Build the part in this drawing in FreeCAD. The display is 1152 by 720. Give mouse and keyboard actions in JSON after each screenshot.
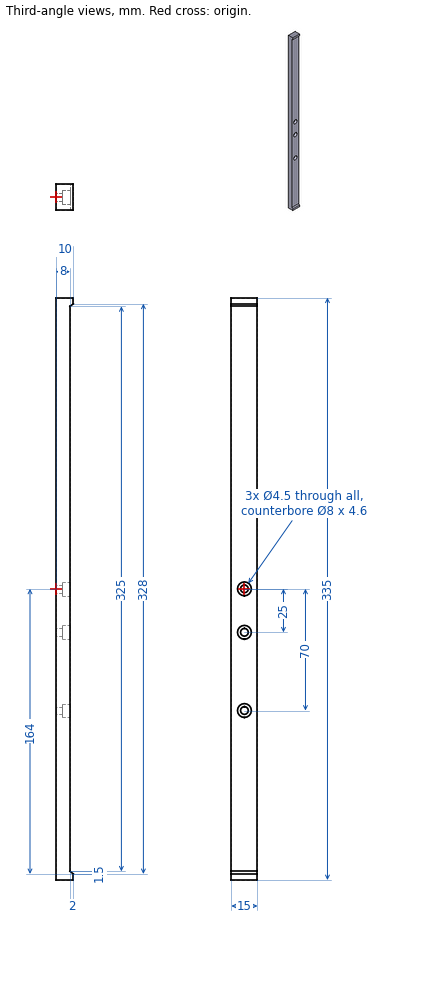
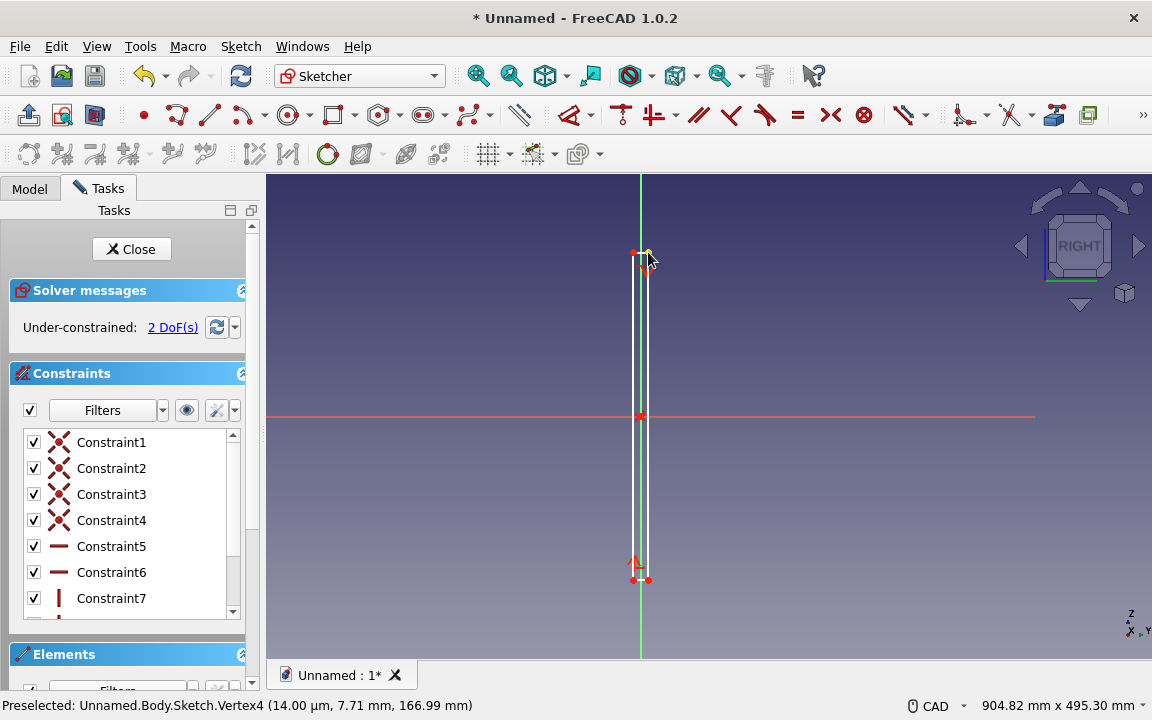
{"action": "scroll", "coordinate": [639, 580], "scroll_direction": "up", "scroll_amount": 5}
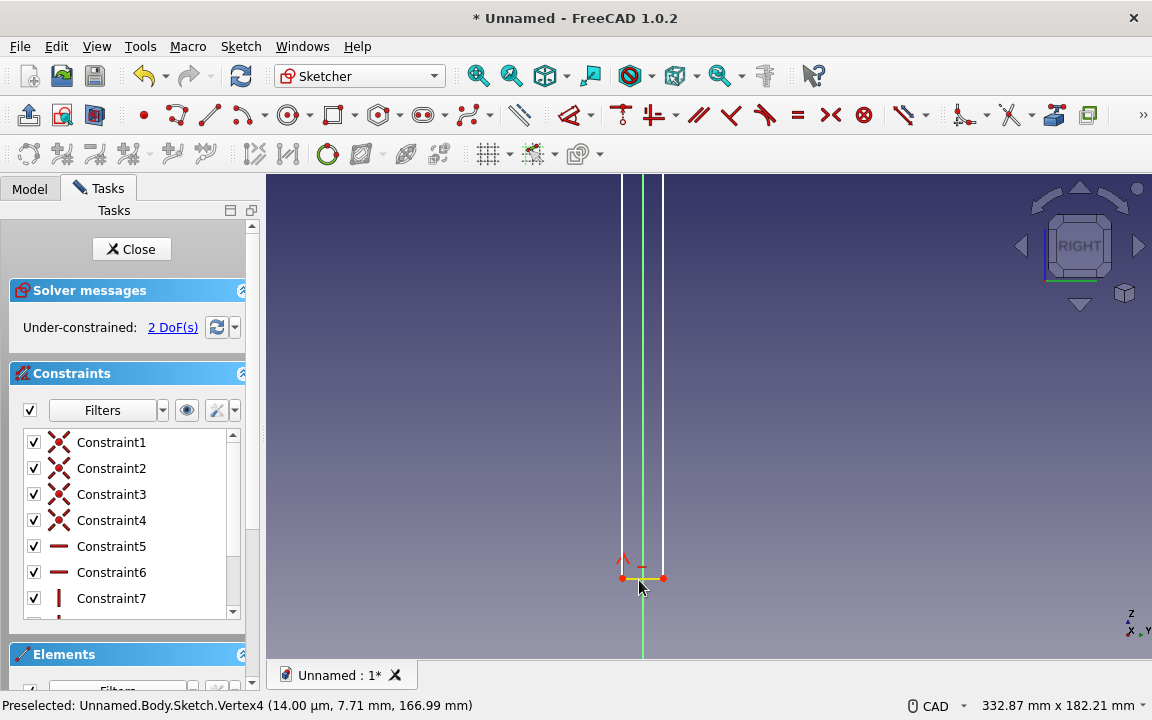
{"action": "left_click", "coordinate": [639, 579]}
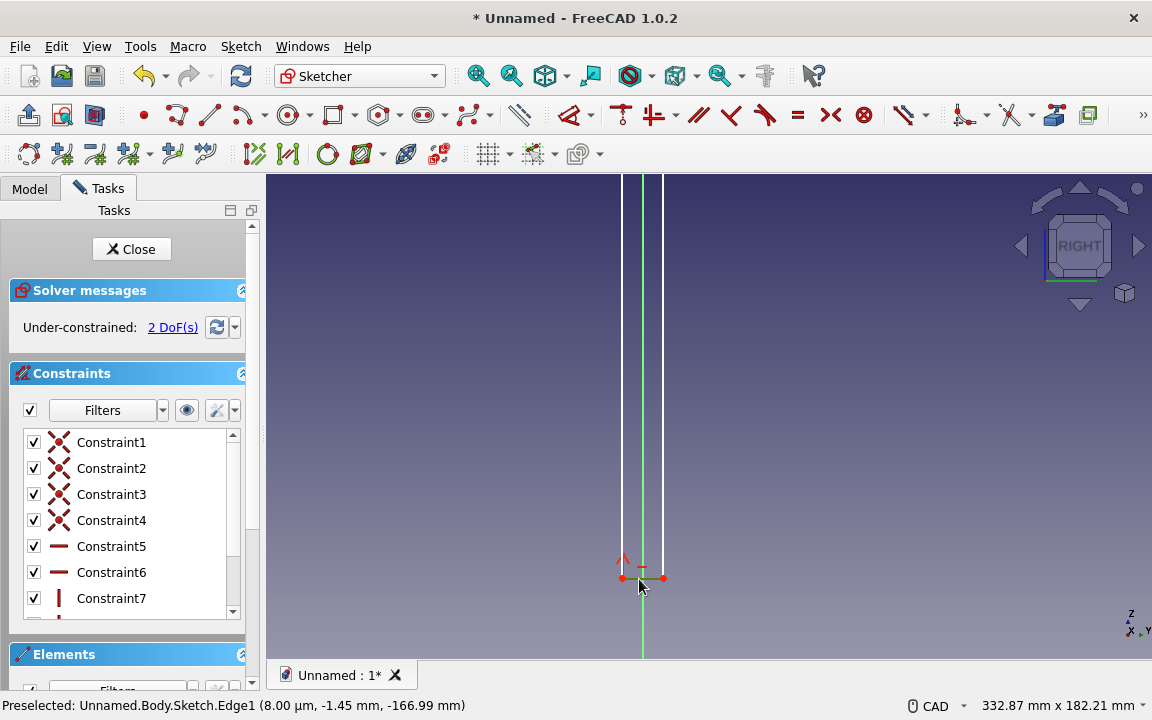
{"action": "key", "text": "l"}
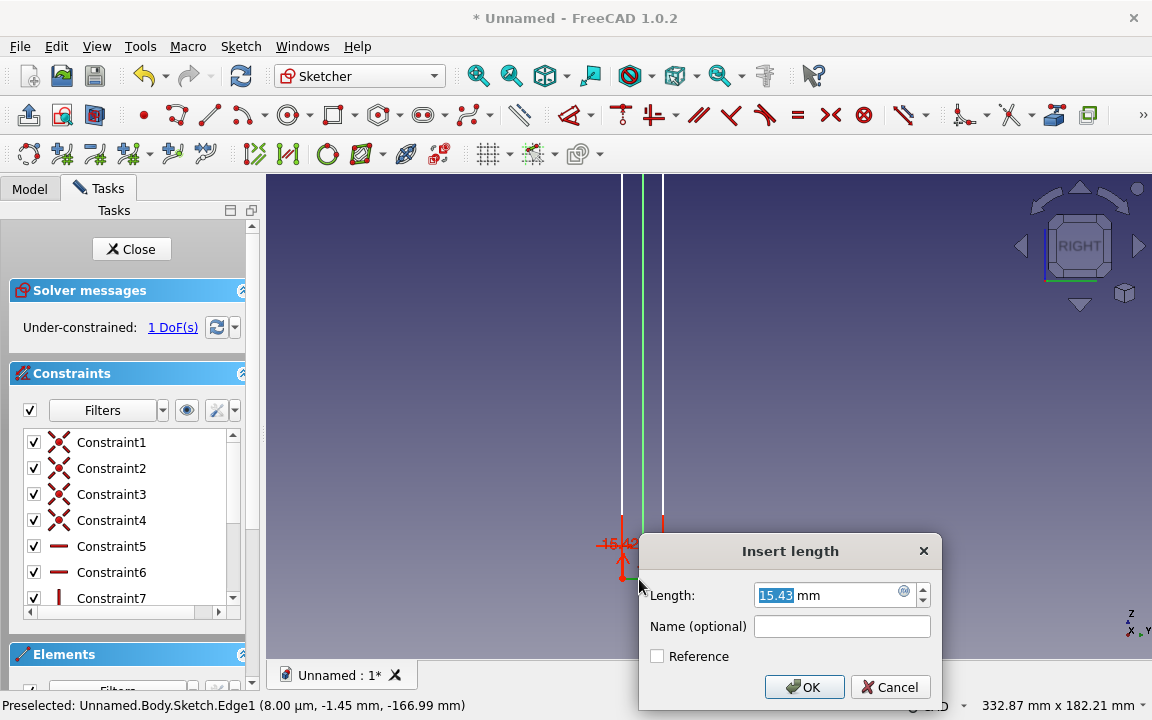
{"action": "type", "text": "15"}
{"action": "key", "text": "Return"}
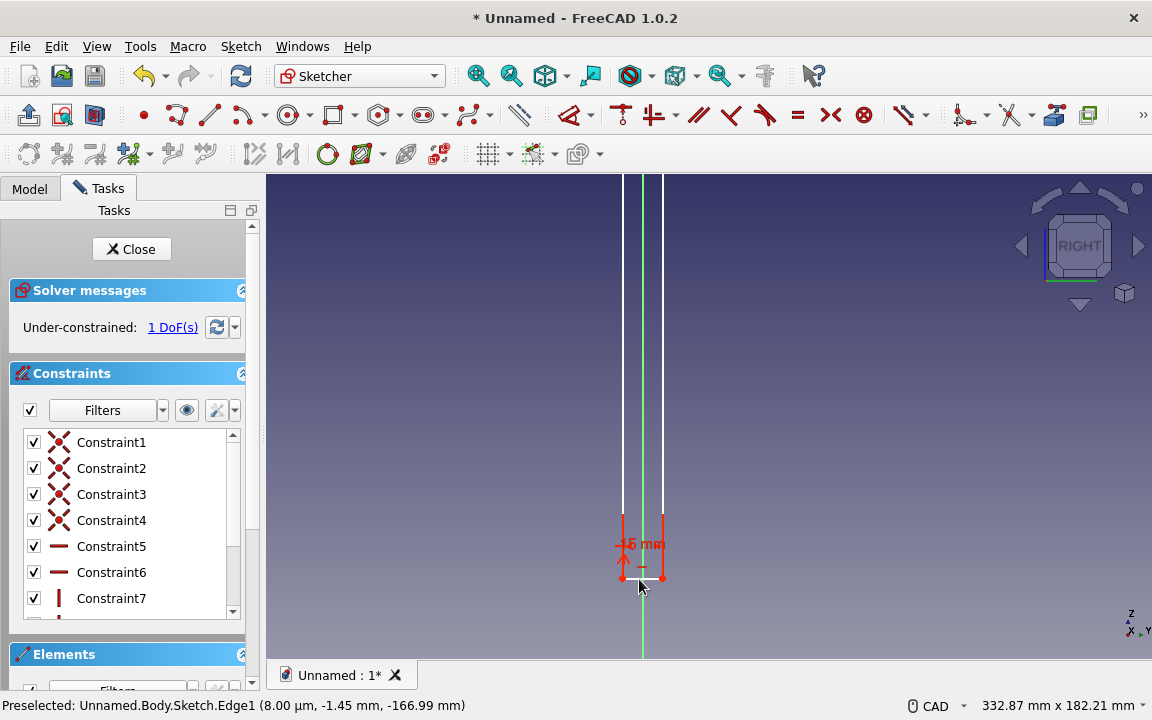
{"action": "left_click", "coordinate": [663, 312]}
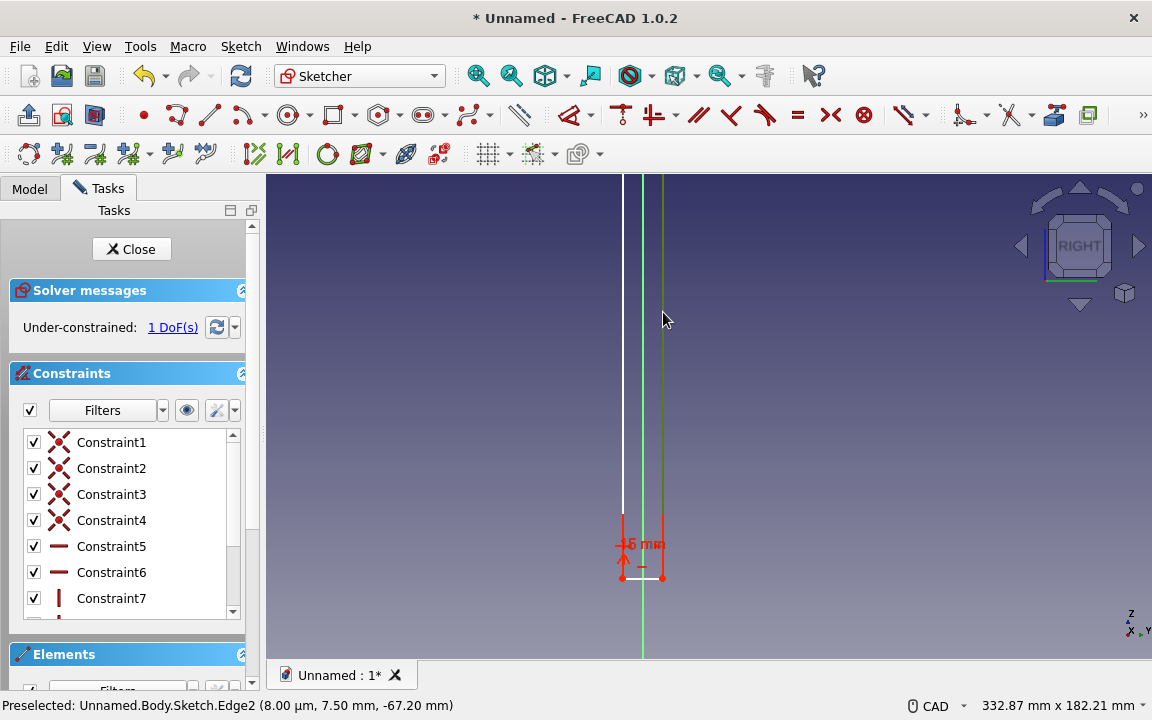
{"action": "key", "text": "i"}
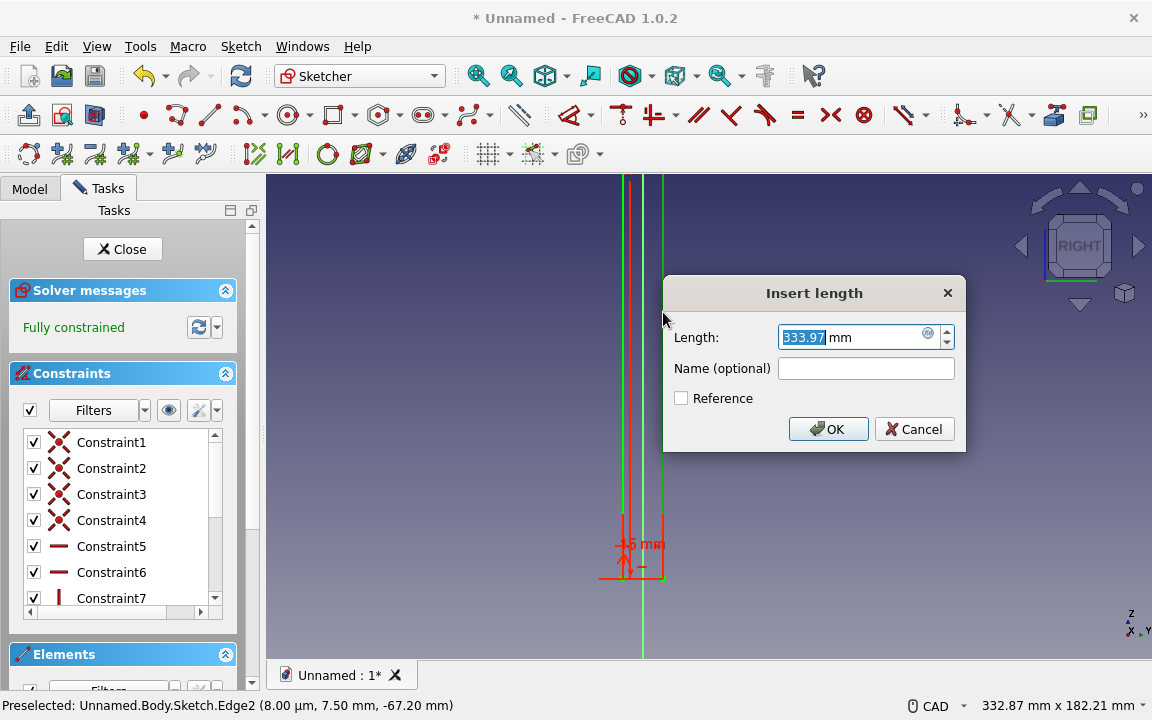
{"action": "type", "text": "335"}
{"action": "key", "text": "Return"}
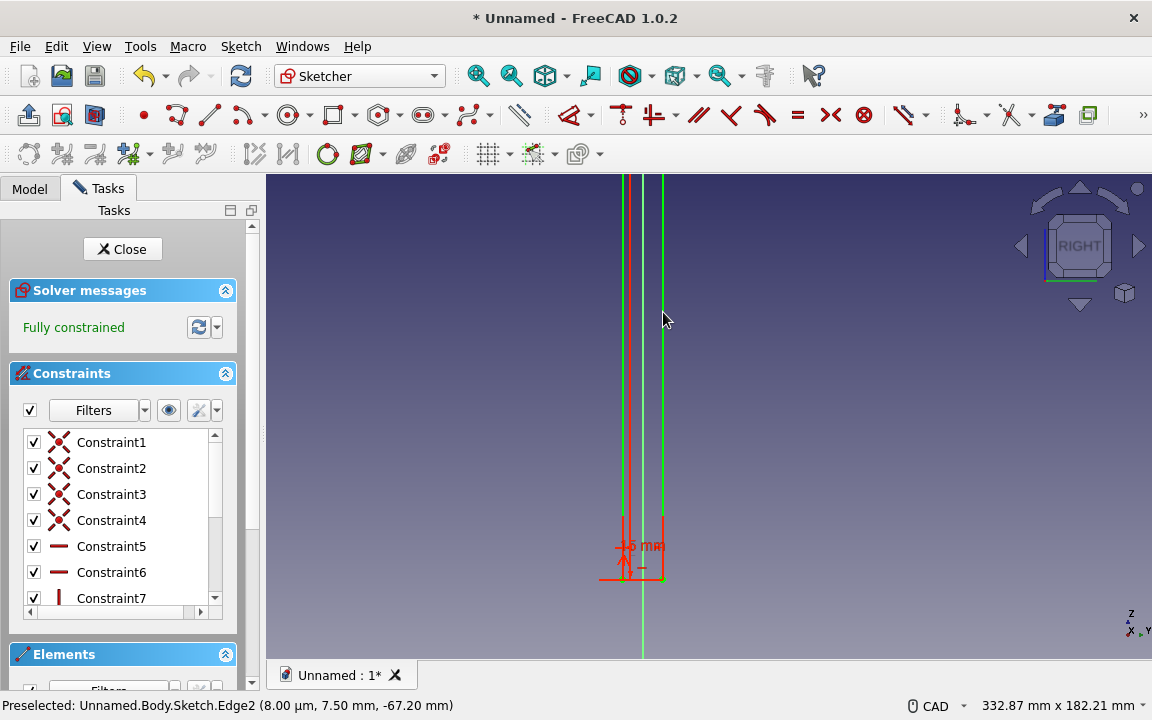
{"action": "left_click", "coordinate": [123, 249]}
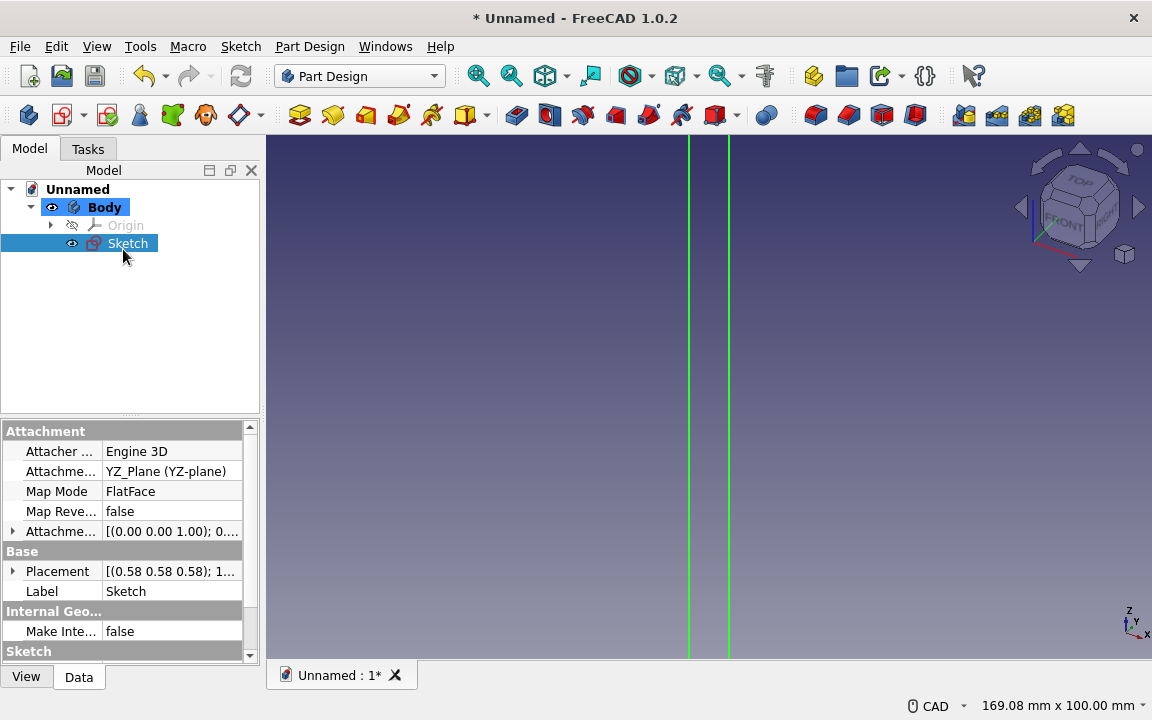
{"action": "left_click", "coordinate": [300, 116]}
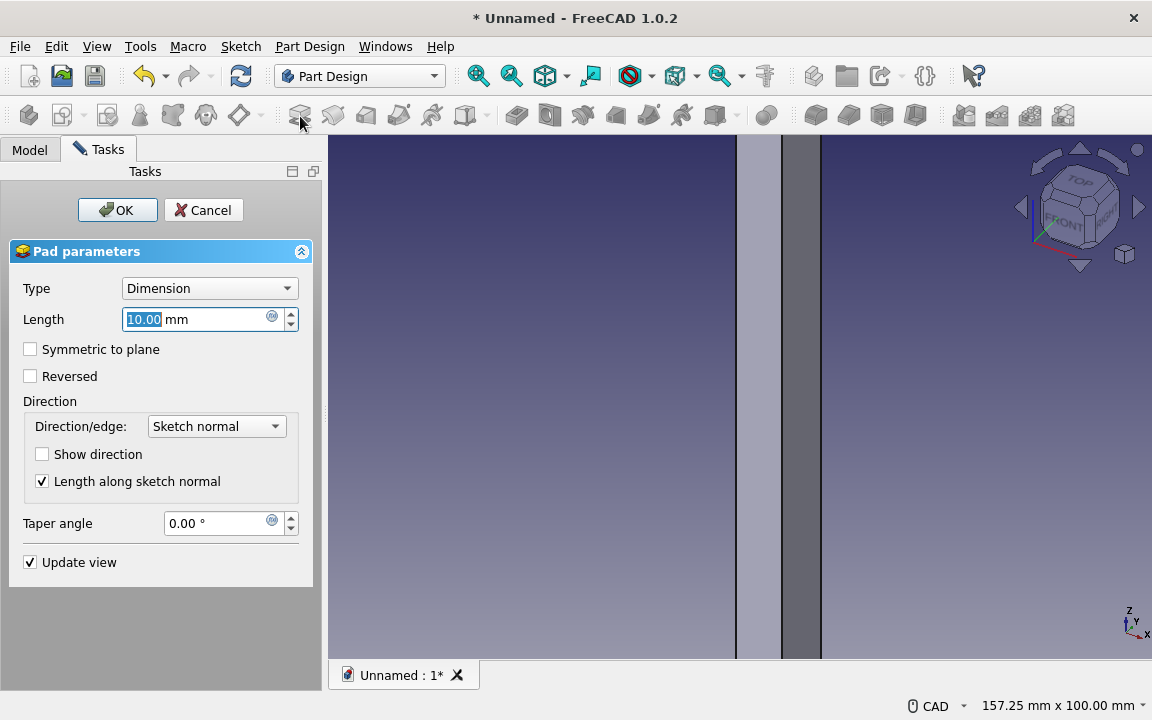
{"action": "type", "text": "10"}
{"action": "key", "text": "Tab"}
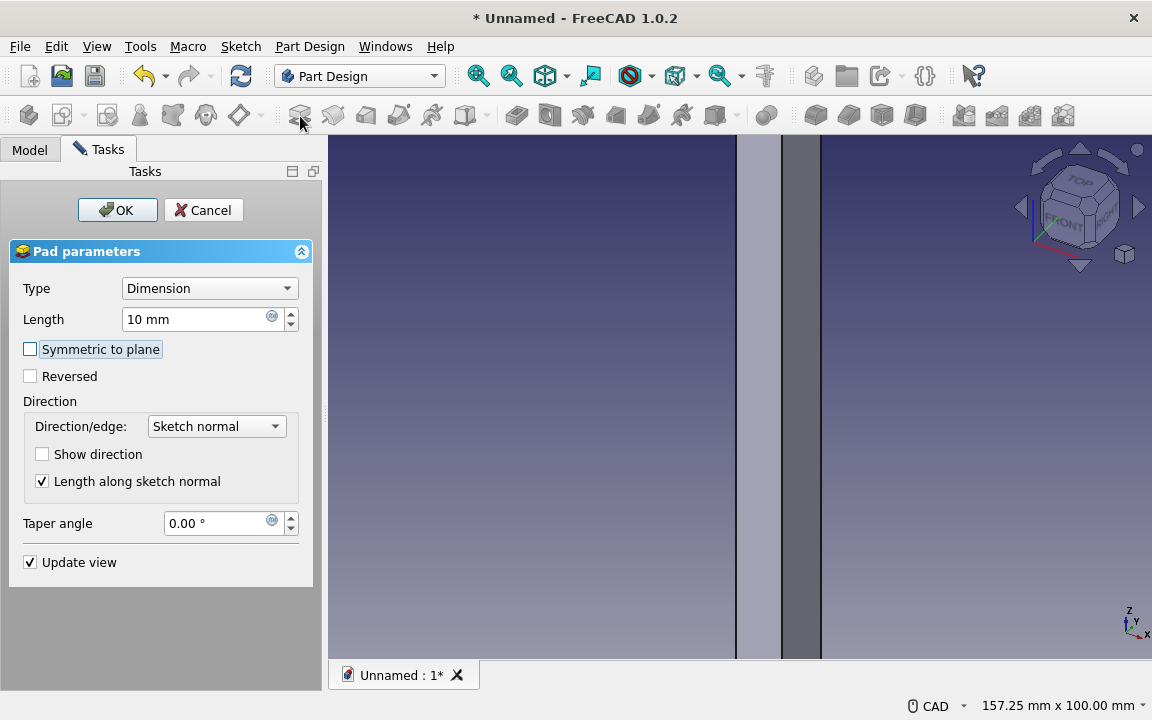
{"action": "left_click", "coordinate": [118, 210]}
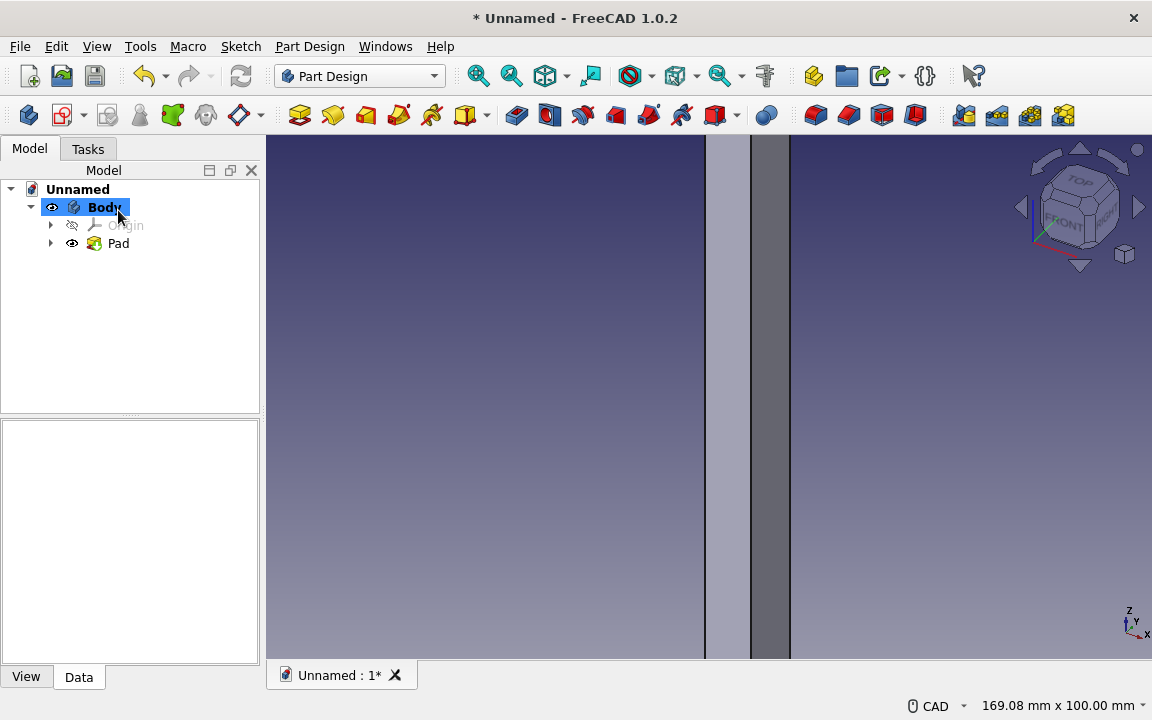
{"action": "left_click", "coordinate": [479, 76]}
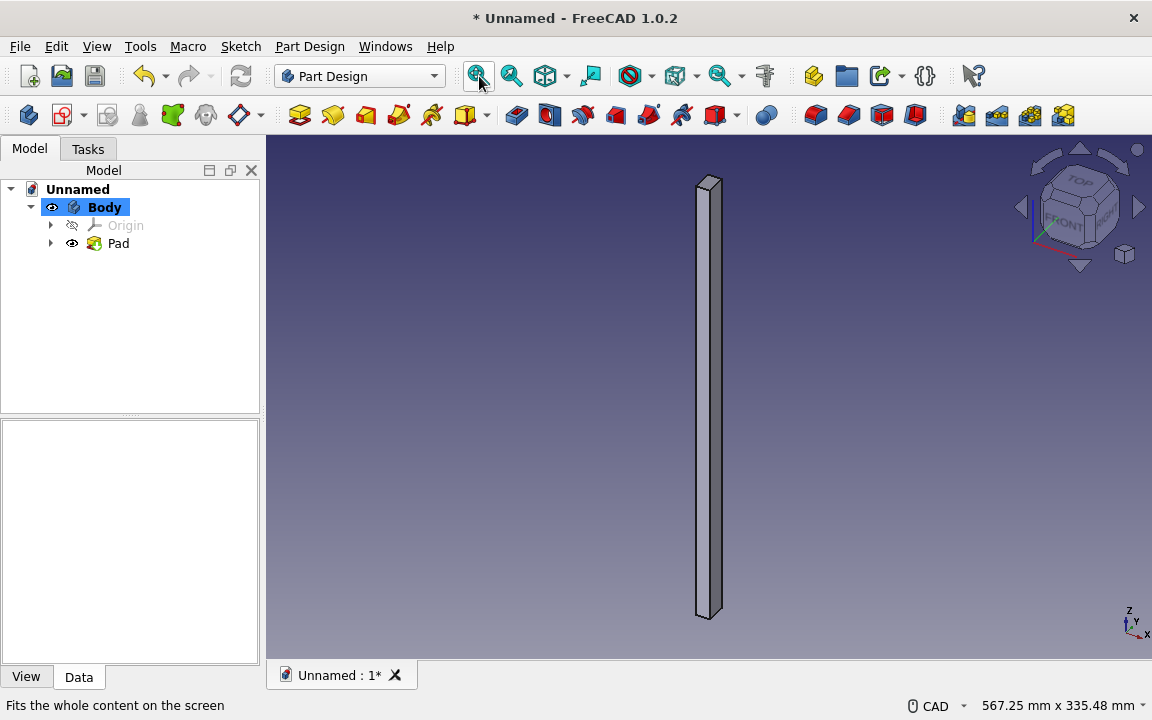
{"action": "key", "text": "0"}